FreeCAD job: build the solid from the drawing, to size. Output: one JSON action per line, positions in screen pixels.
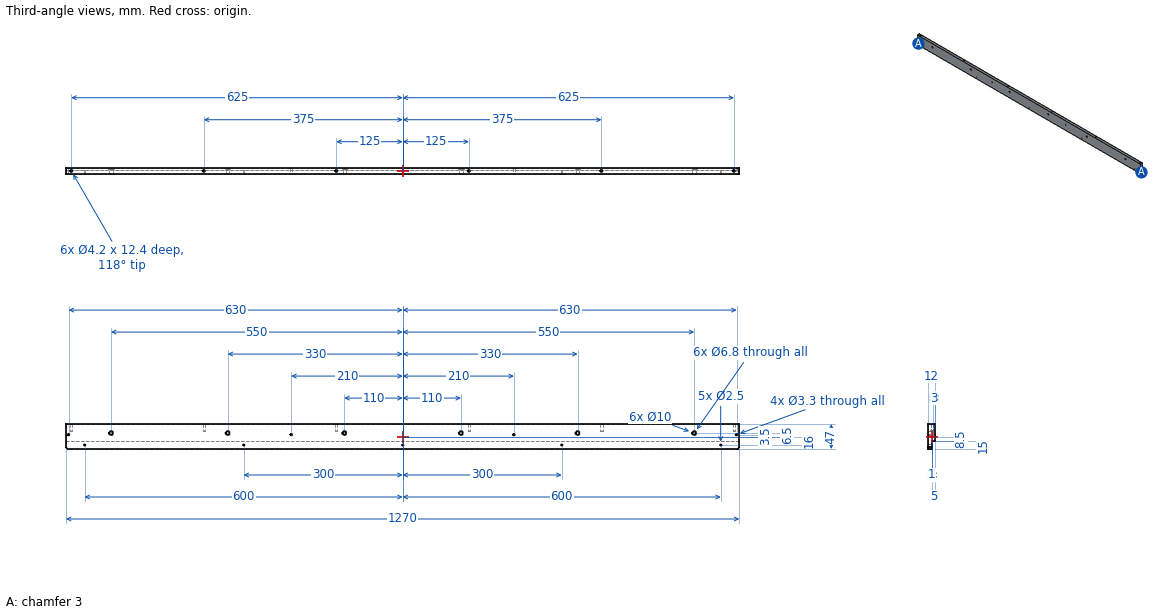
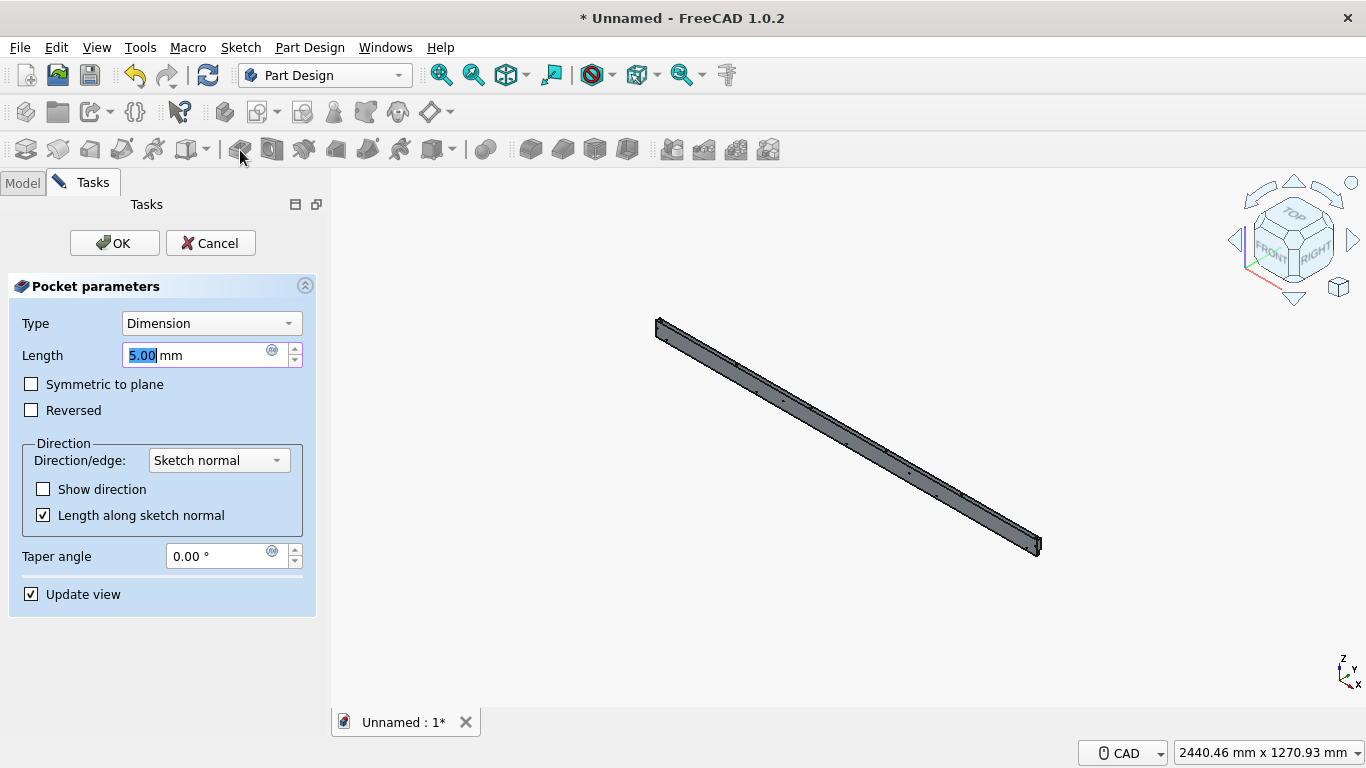
{"action": "left_click", "coordinate": [212, 324]}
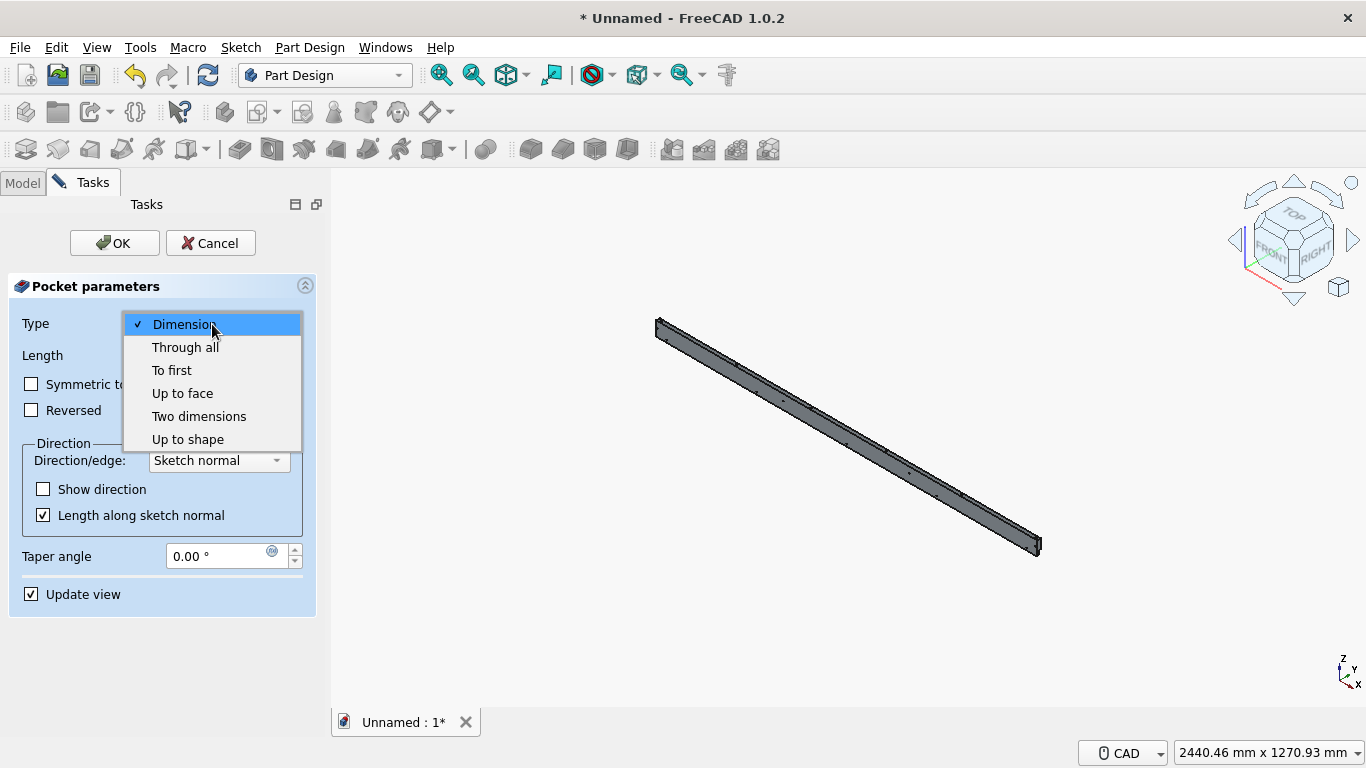
{"action": "left_click", "coordinate": [212, 348]}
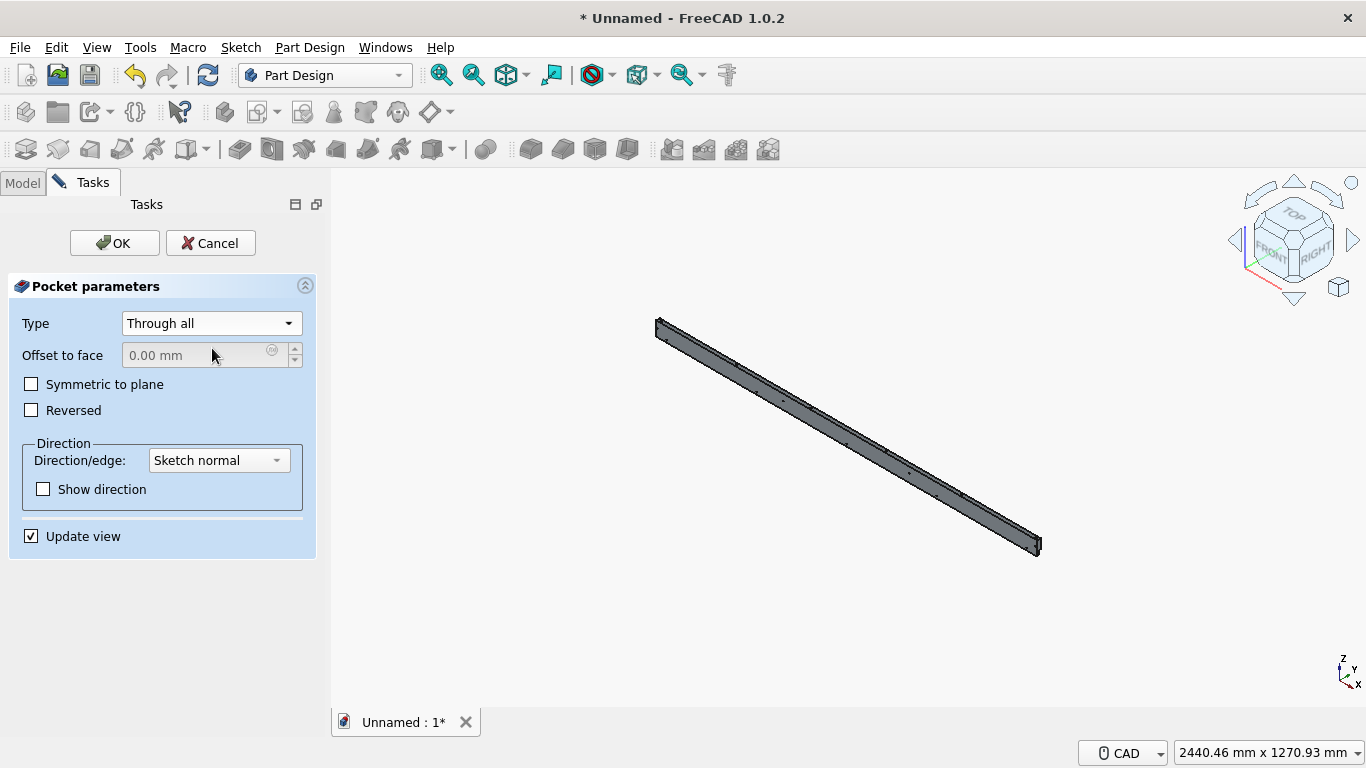
{"action": "left_click", "coordinate": [115, 243]}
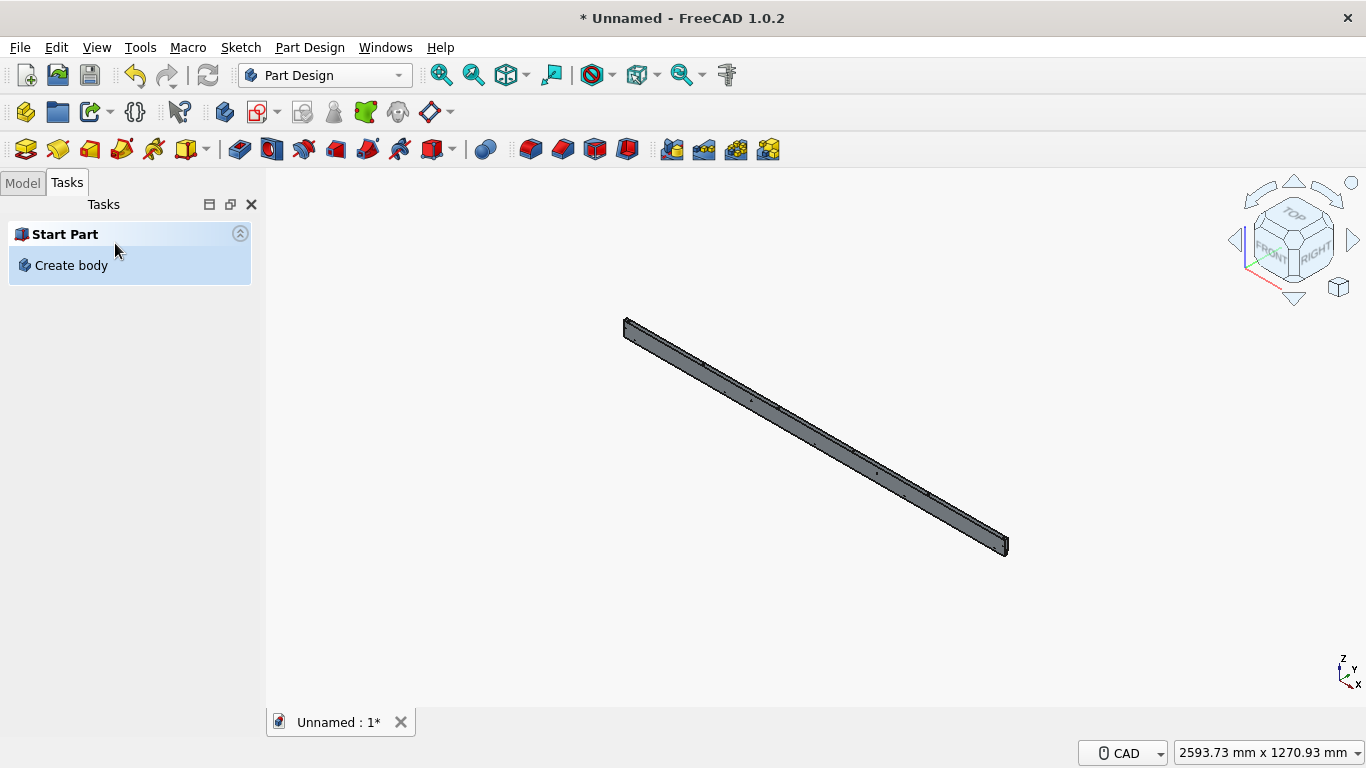
{"action": "left_click", "coordinate": [442, 76]}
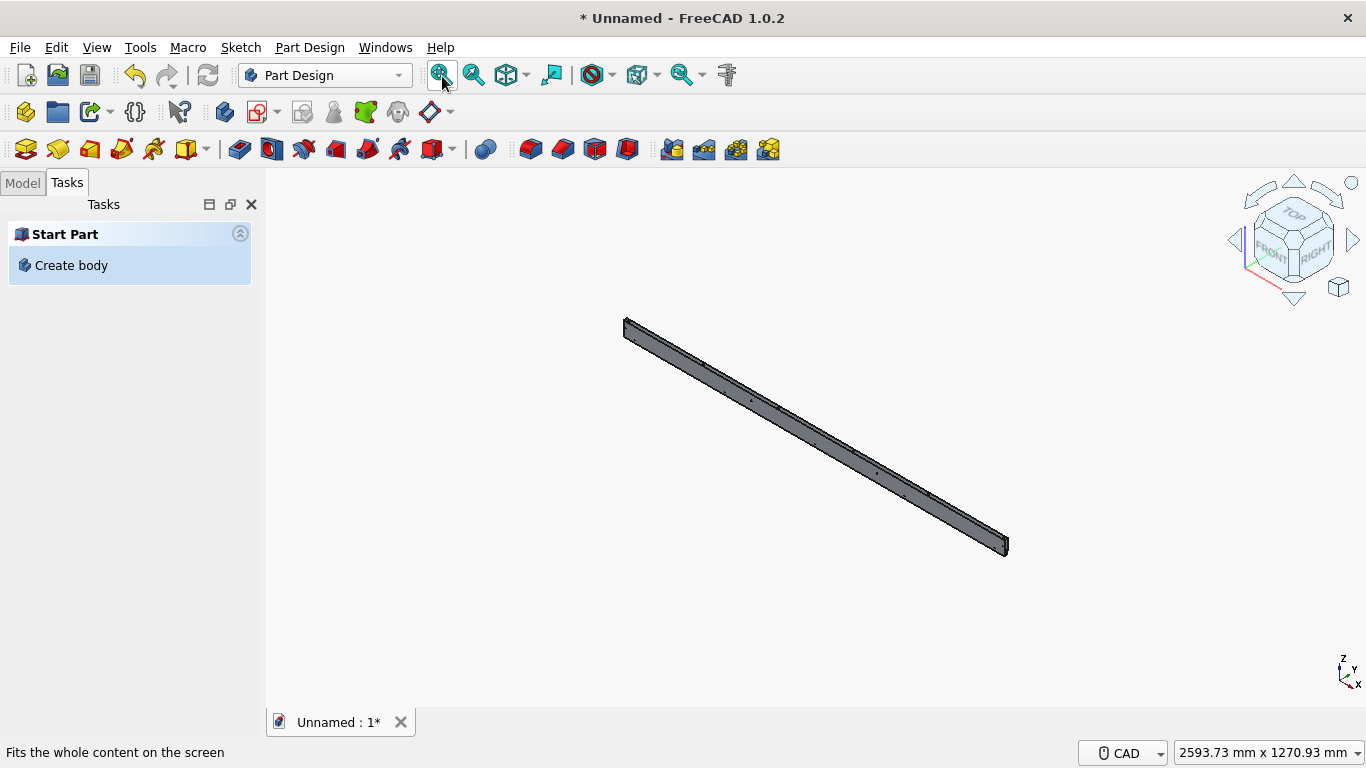
{"action": "left_click", "coordinate": [977, 534]}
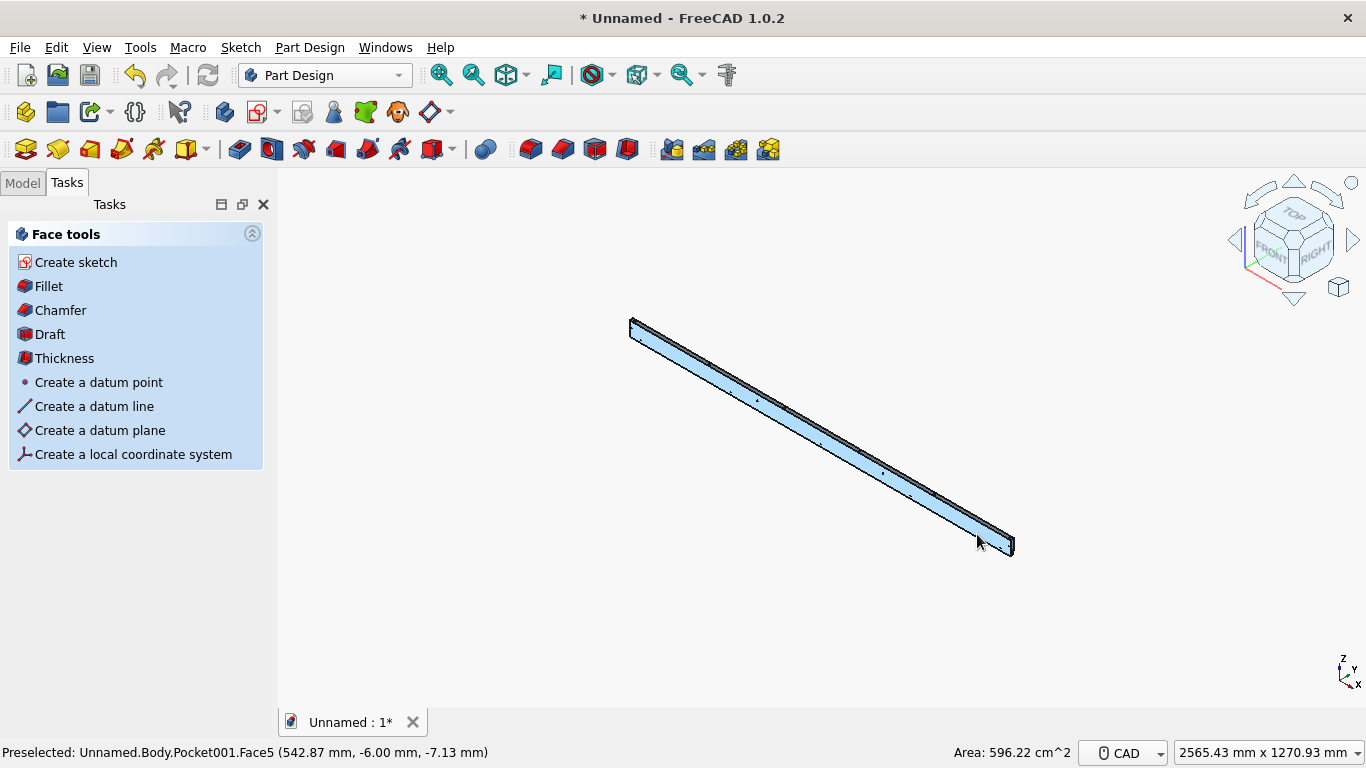
{"action": "left_click", "coordinate": [258, 112]}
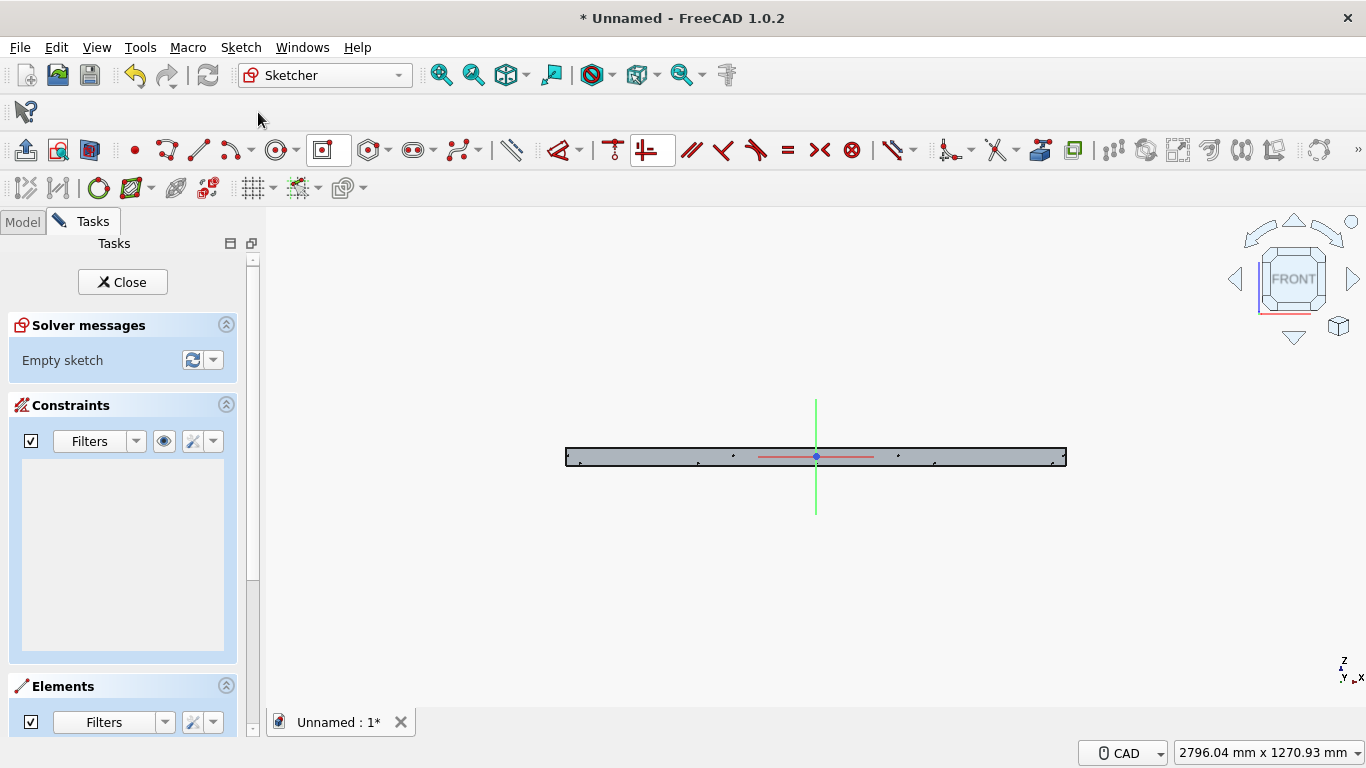
{"action": "scroll", "coordinate": [955, 451], "scroll_direction": "up", "scroll_amount": 2}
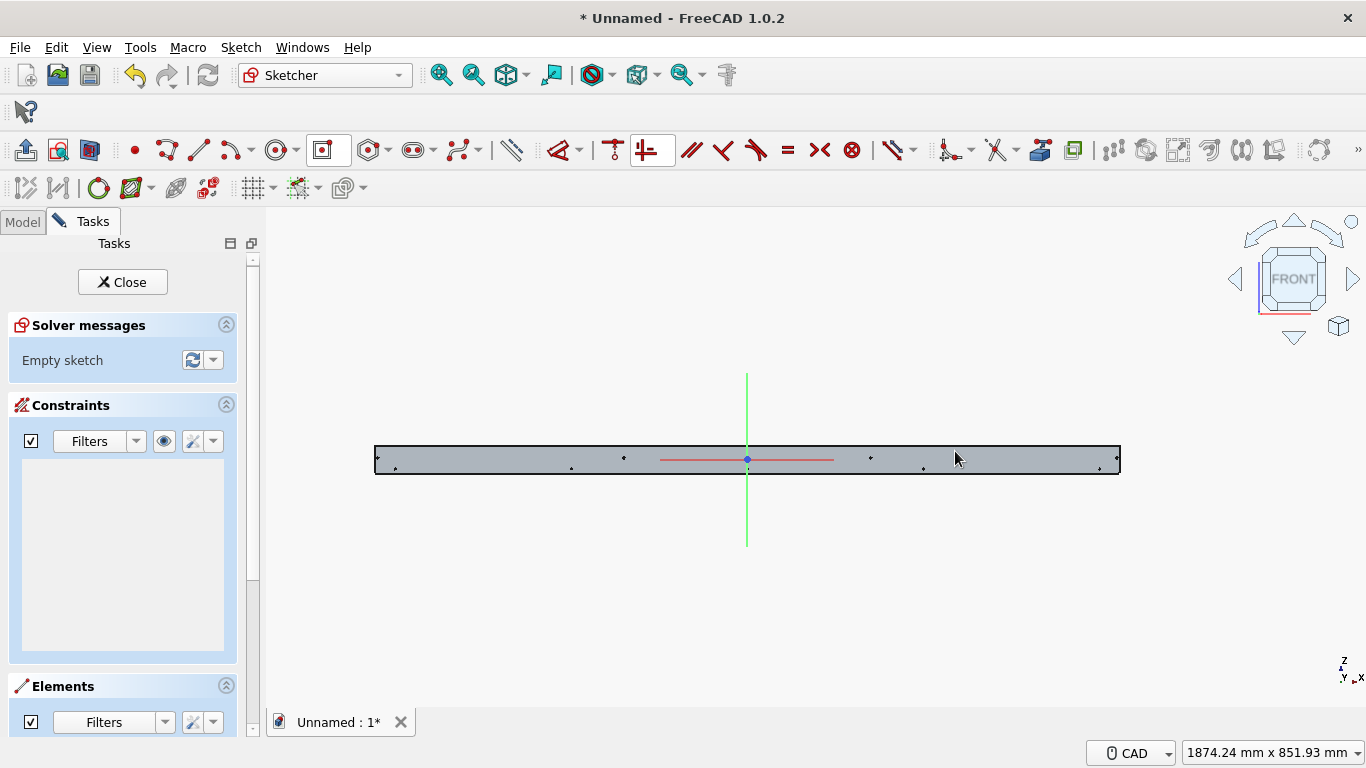
{"action": "left_click", "coordinate": [276, 150]}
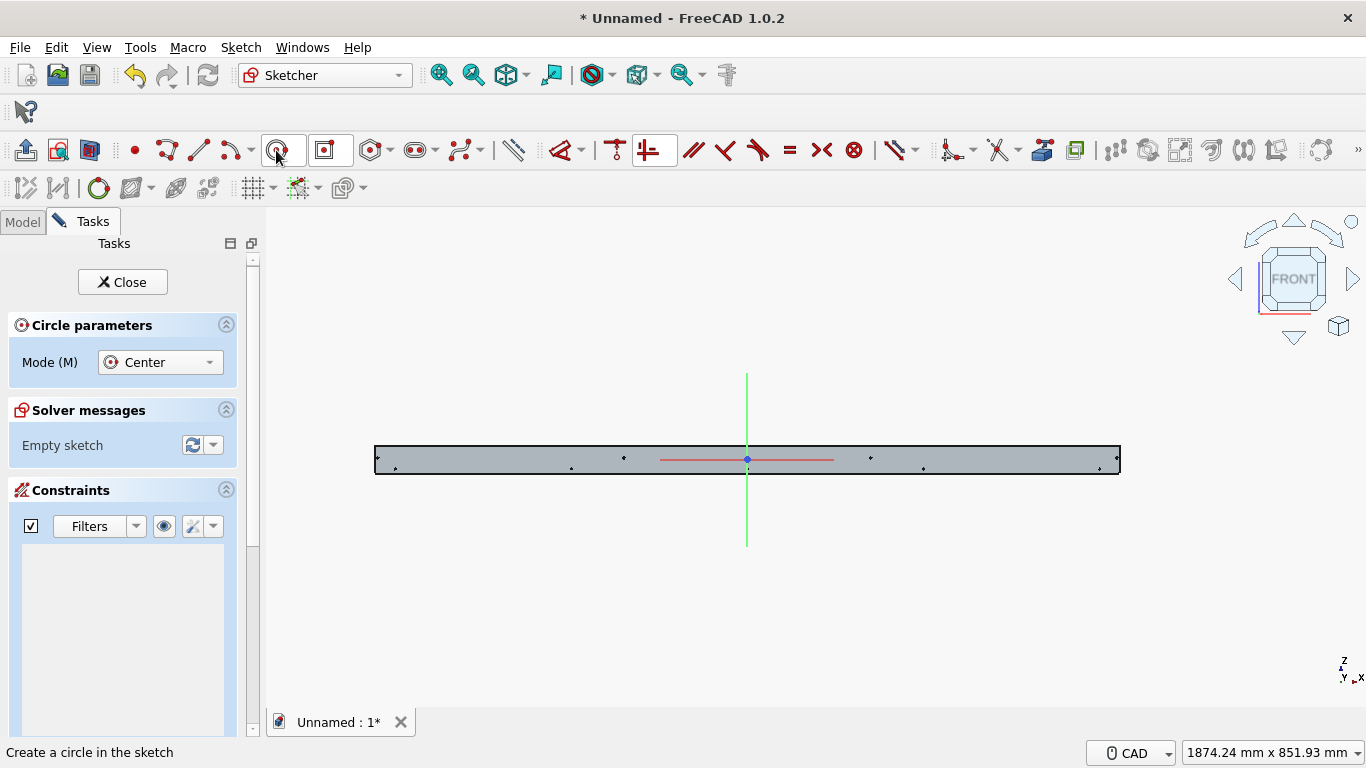
{"action": "scroll", "coordinate": [1070, 456], "scroll_direction": "up", "scroll_amount": 13}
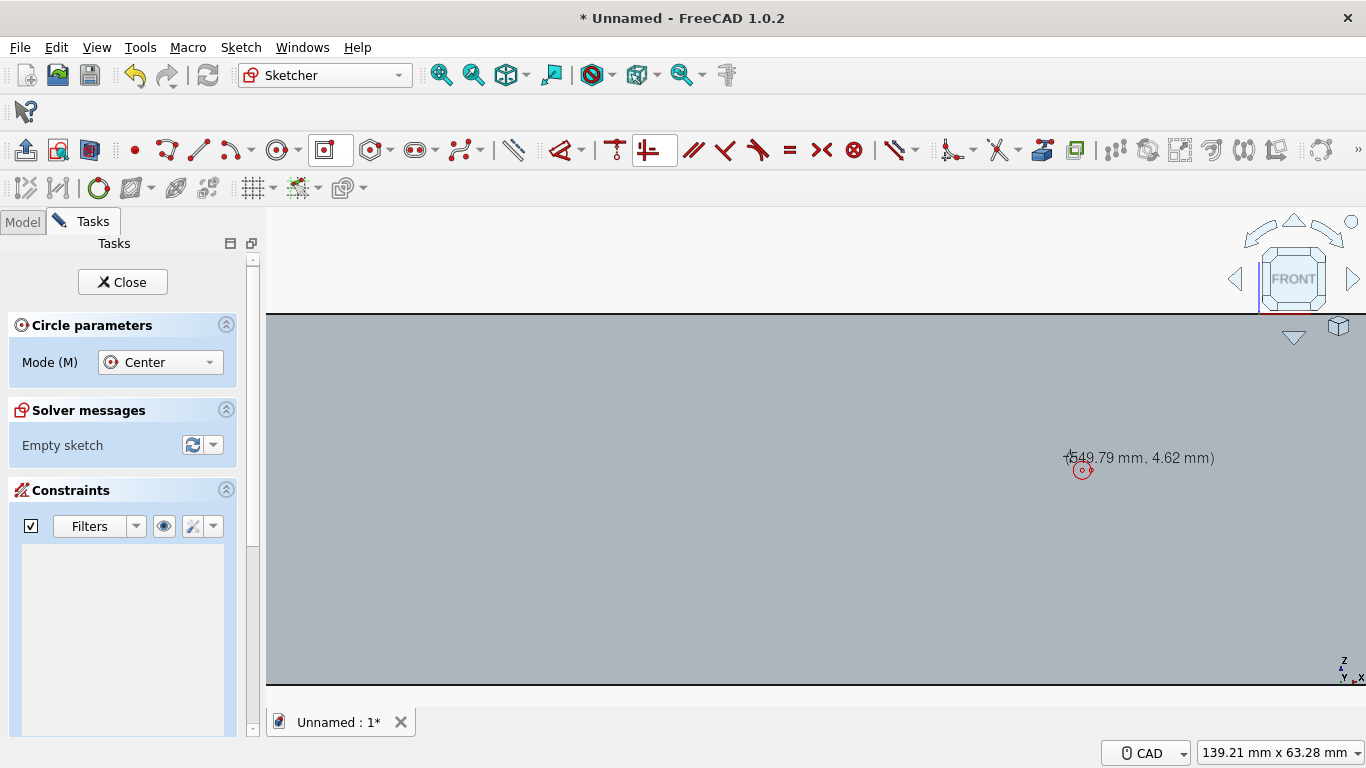
{"action": "scroll", "coordinate": [1071, 457], "scroll_direction": "down", "scroll_amount": 13}